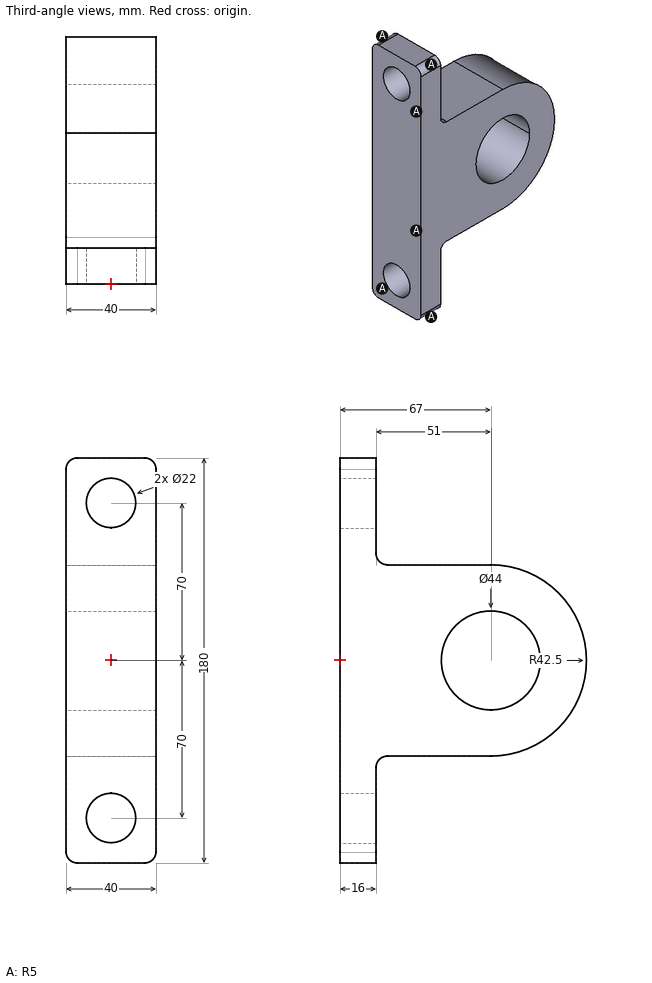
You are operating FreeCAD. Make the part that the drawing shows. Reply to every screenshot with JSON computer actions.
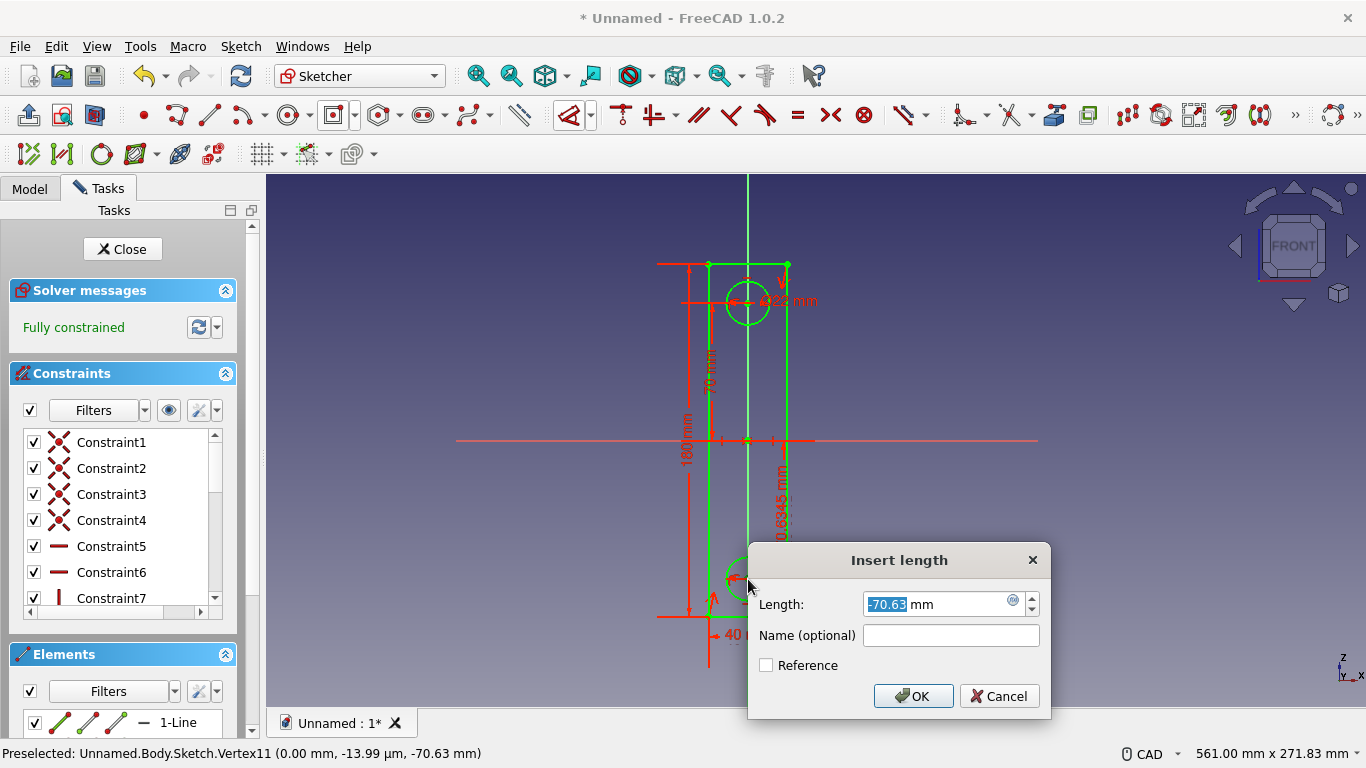
{"action": "type", "text": "-70"}
{"action": "key", "text": "Return"}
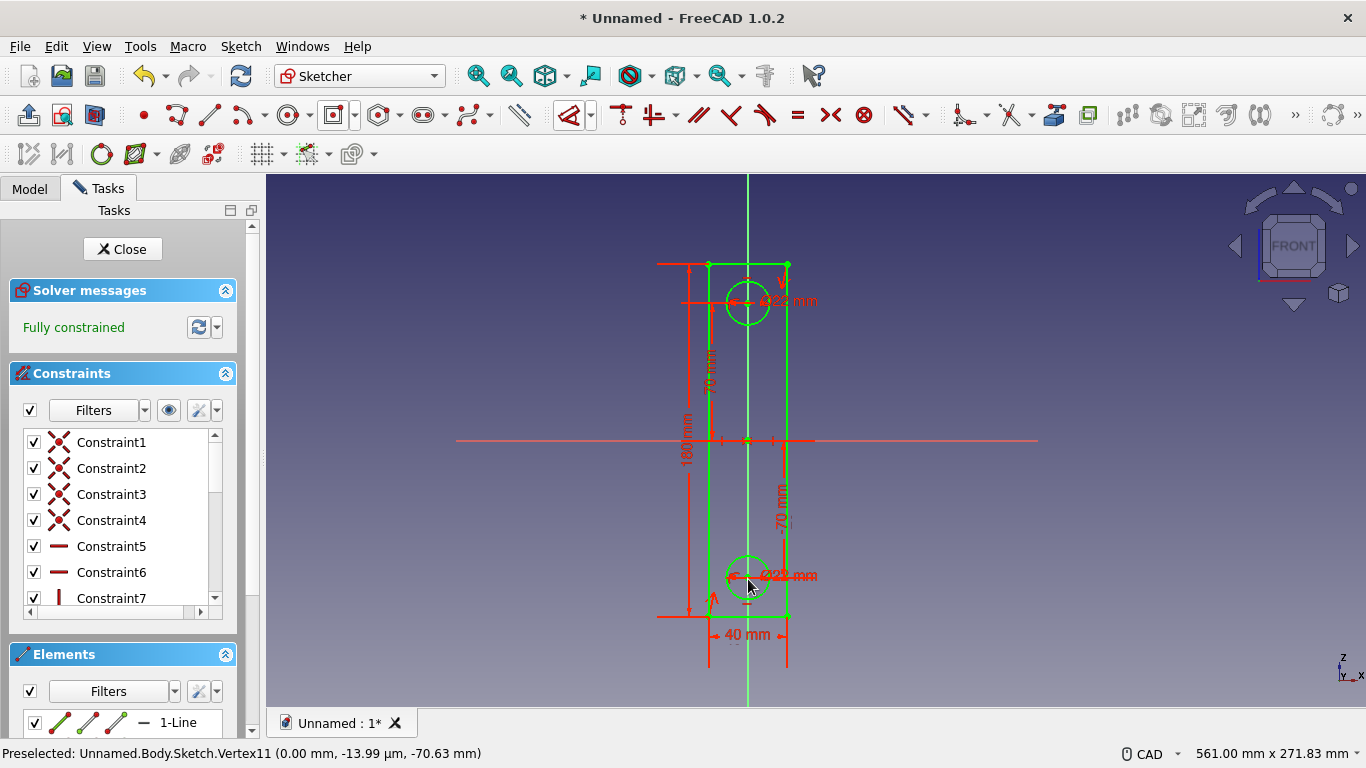
{"action": "left_click", "coordinate": [123, 249]}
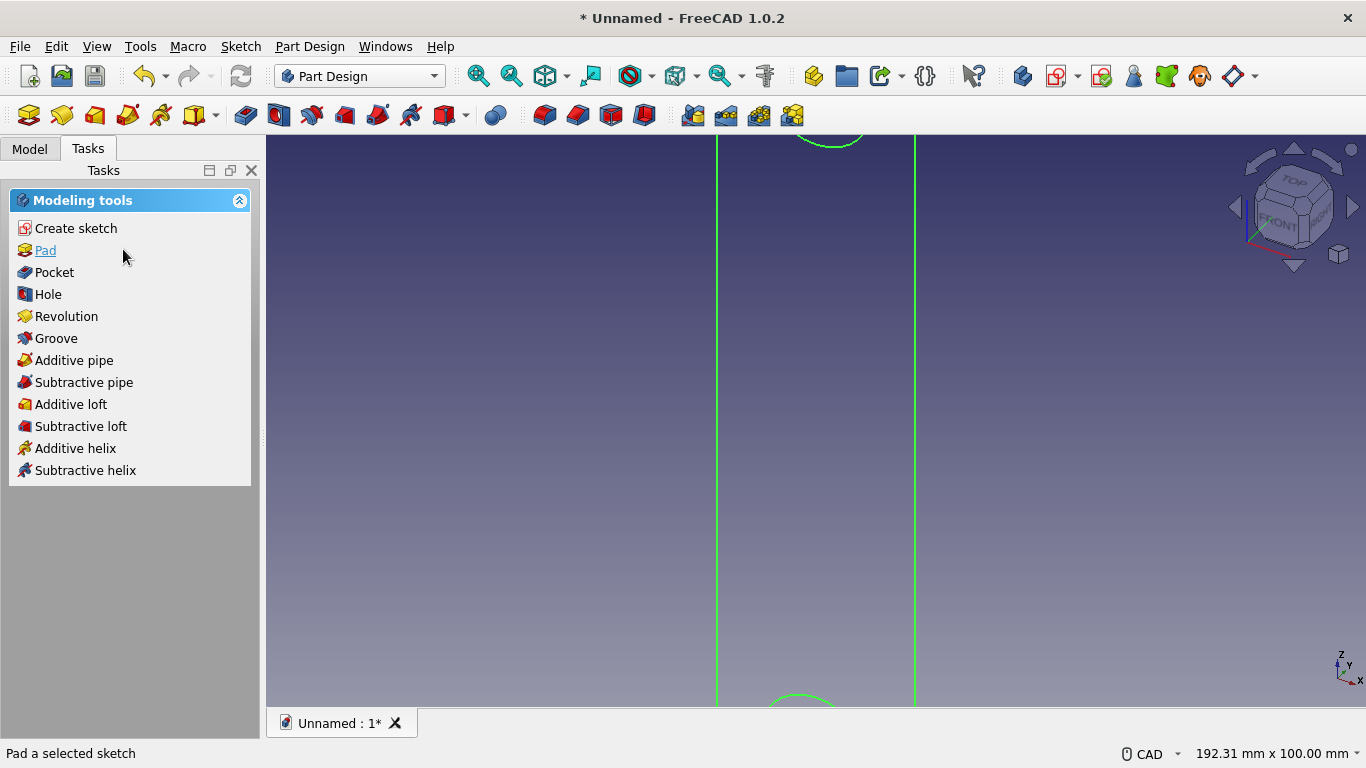
{"action": "left_click", "coordinate": [29, 116]}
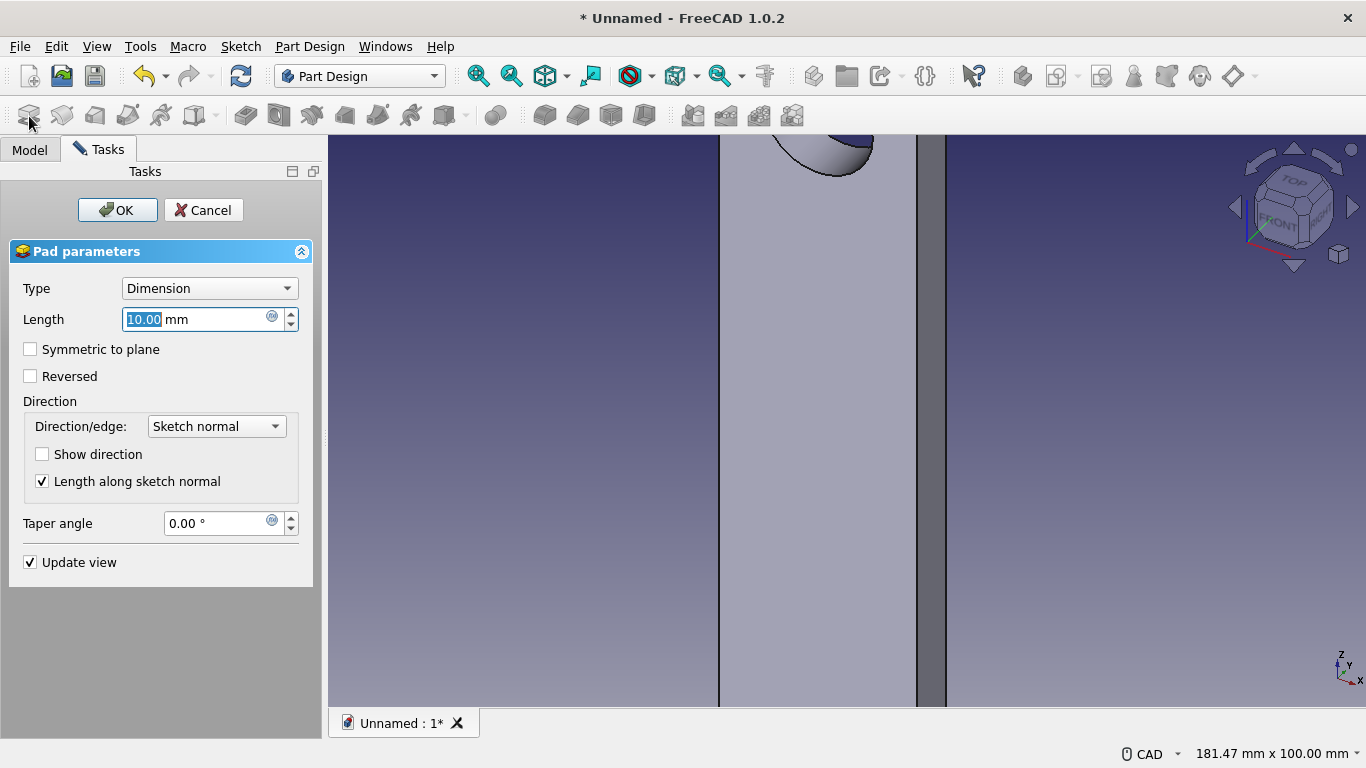
{"action": "type", "text": "16"}
{"action": "key", "text": "Tab"}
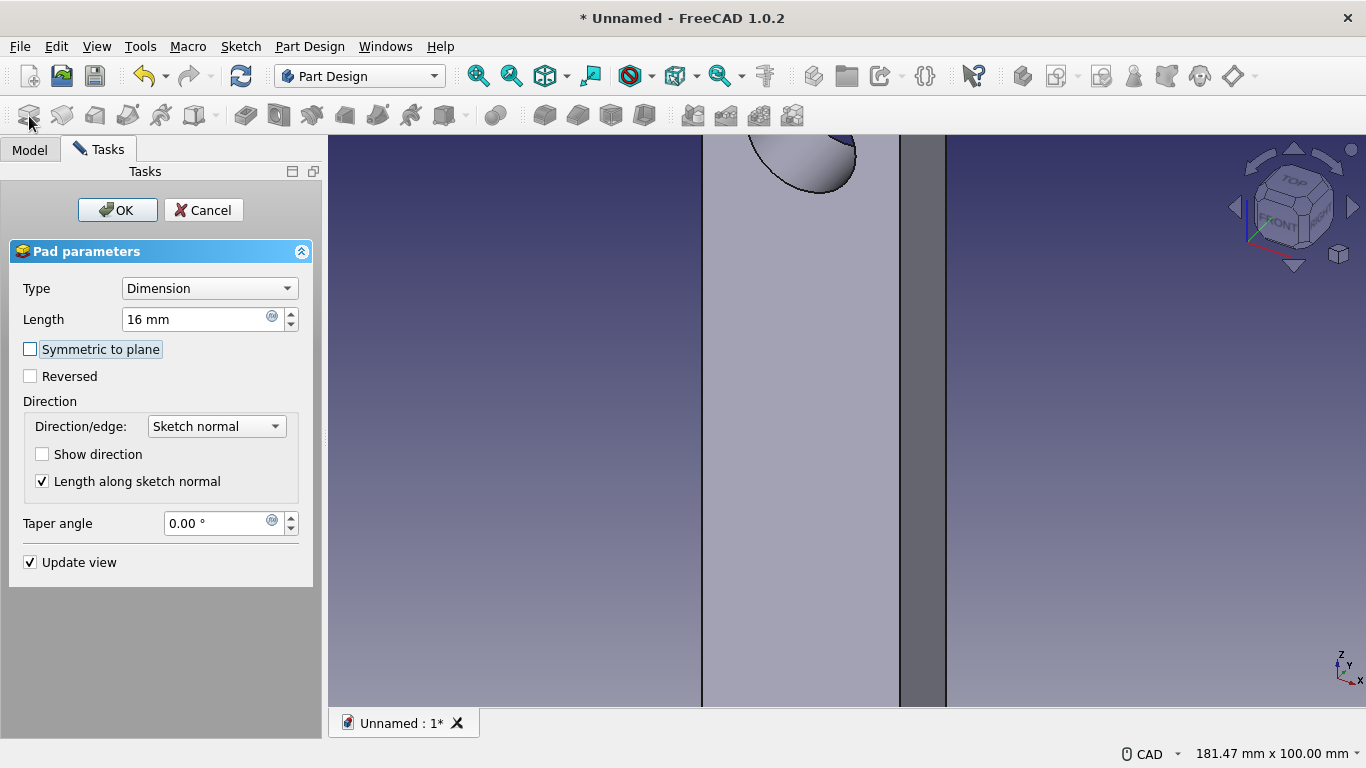
{"action": "left_click", "coordinate": [31, 376]}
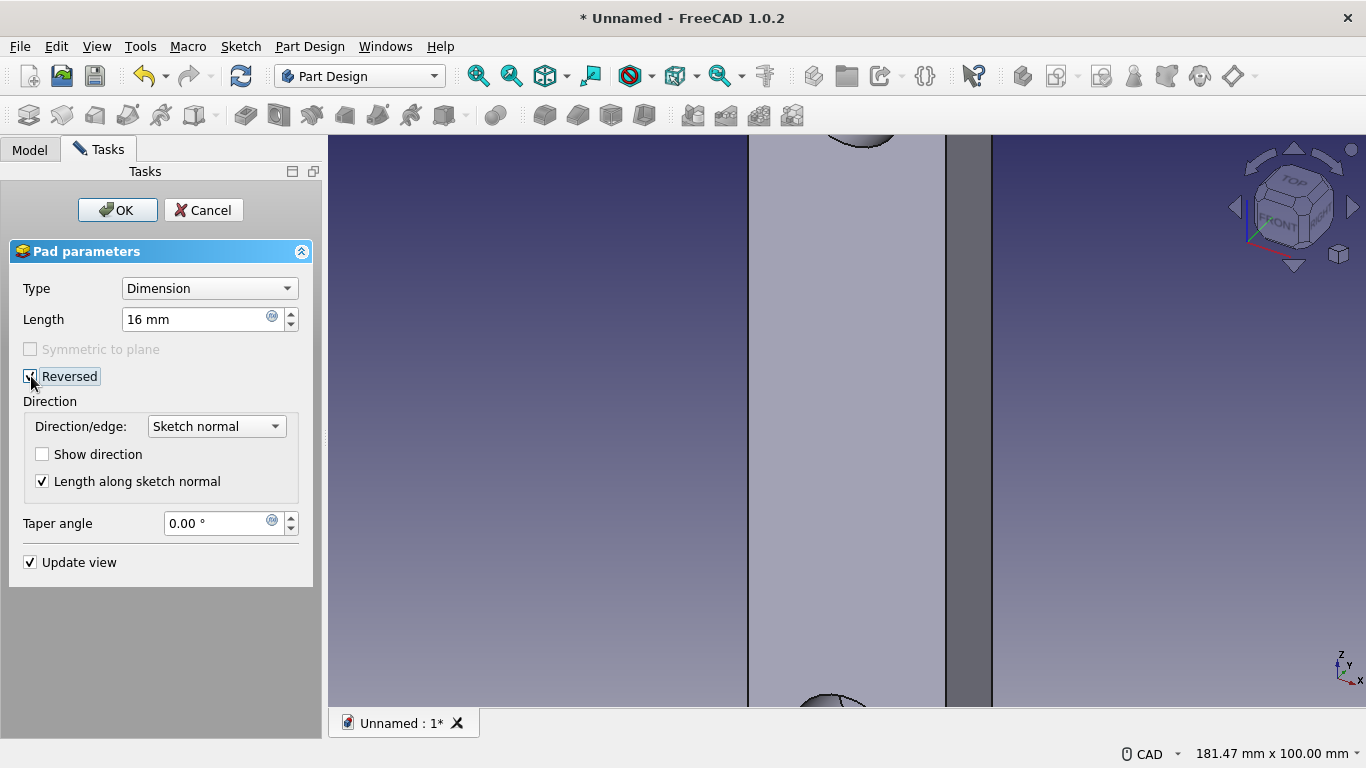
{"action": "left_click", "coordinate": [118, 210]}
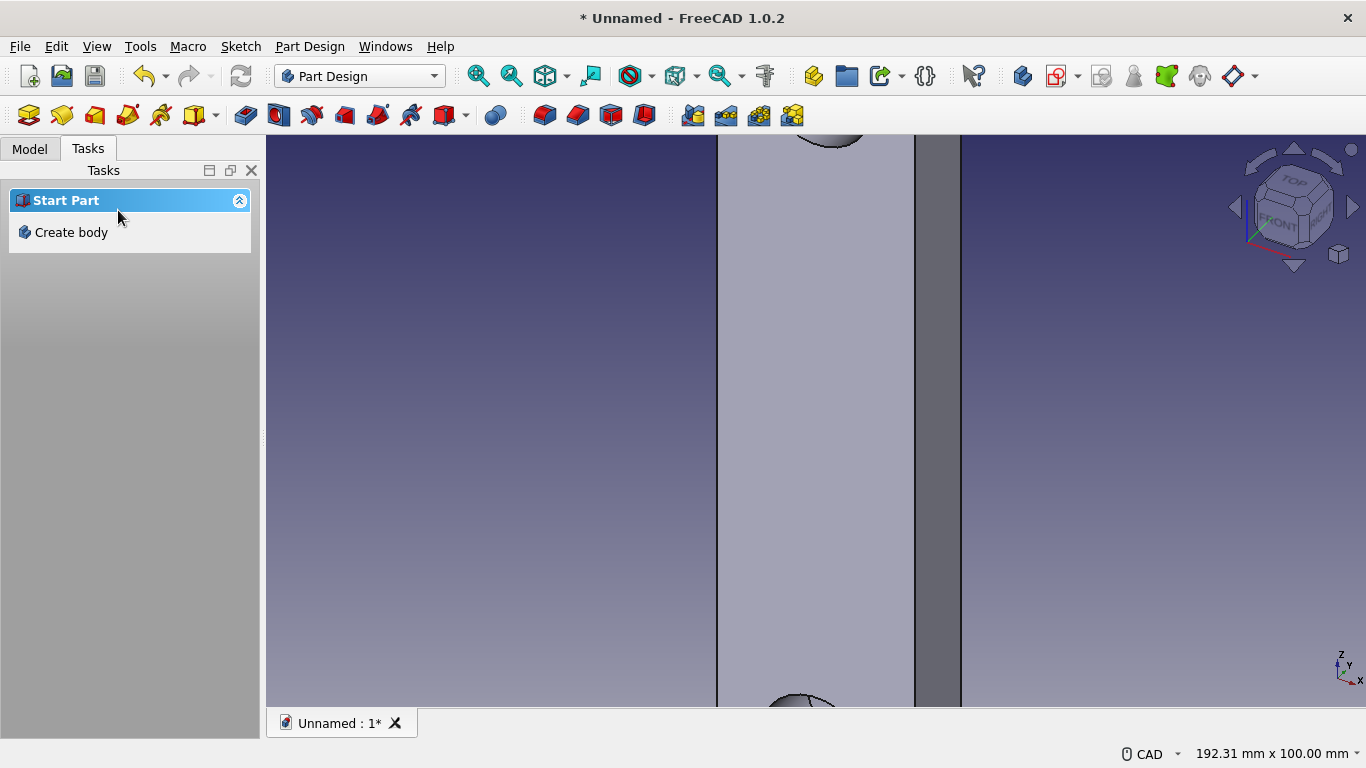
{"action": "left_click", "coordinate": [479, 76]}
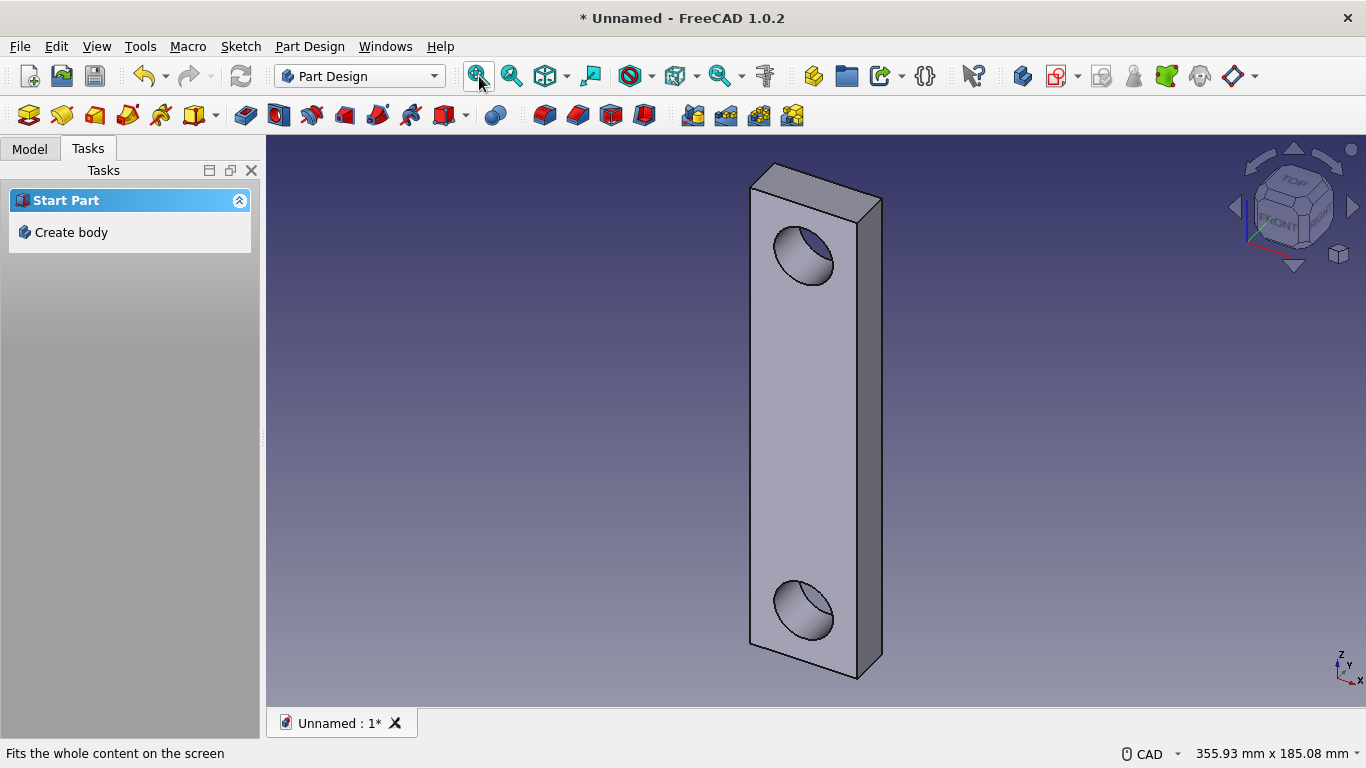
{"action": "left_click", "coordinate": [1056, 76]}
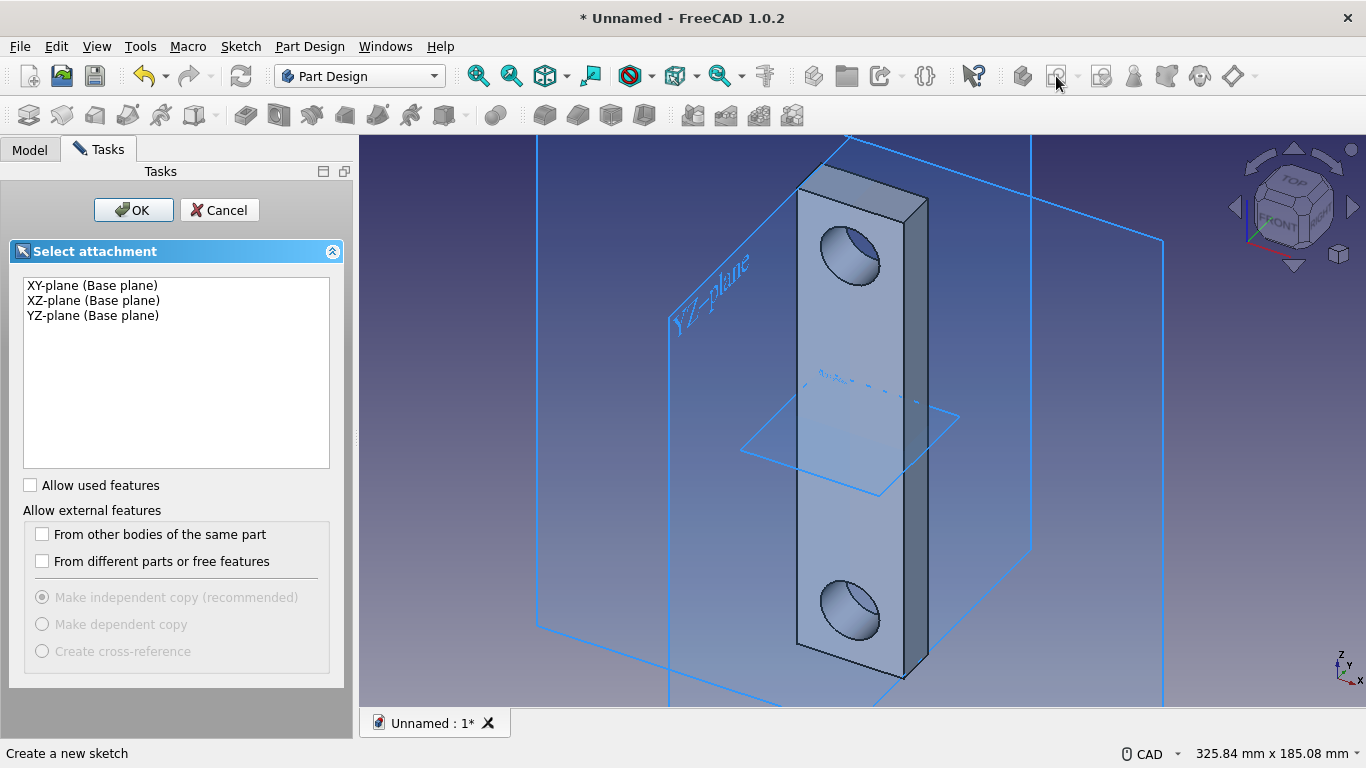
{"action": "left_click", "coordinate": [84, 316]}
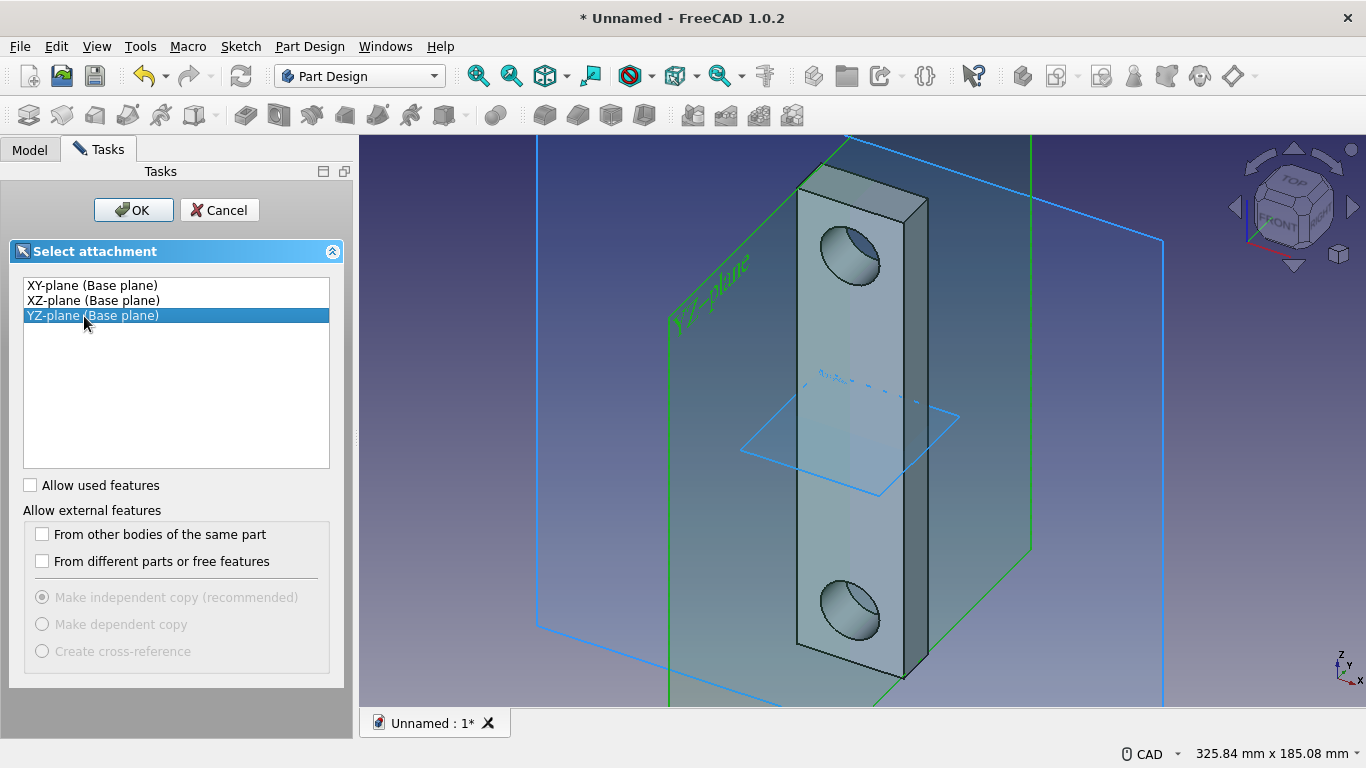
{"action": "left_click", "coordinate": [134, 210]}